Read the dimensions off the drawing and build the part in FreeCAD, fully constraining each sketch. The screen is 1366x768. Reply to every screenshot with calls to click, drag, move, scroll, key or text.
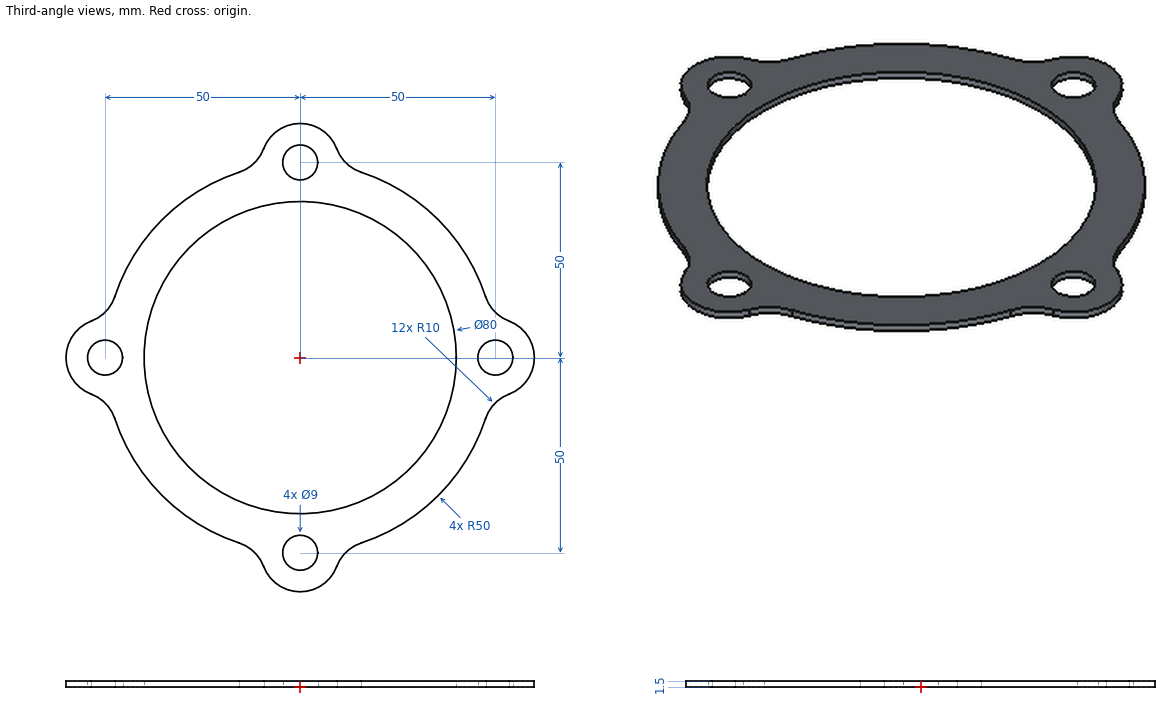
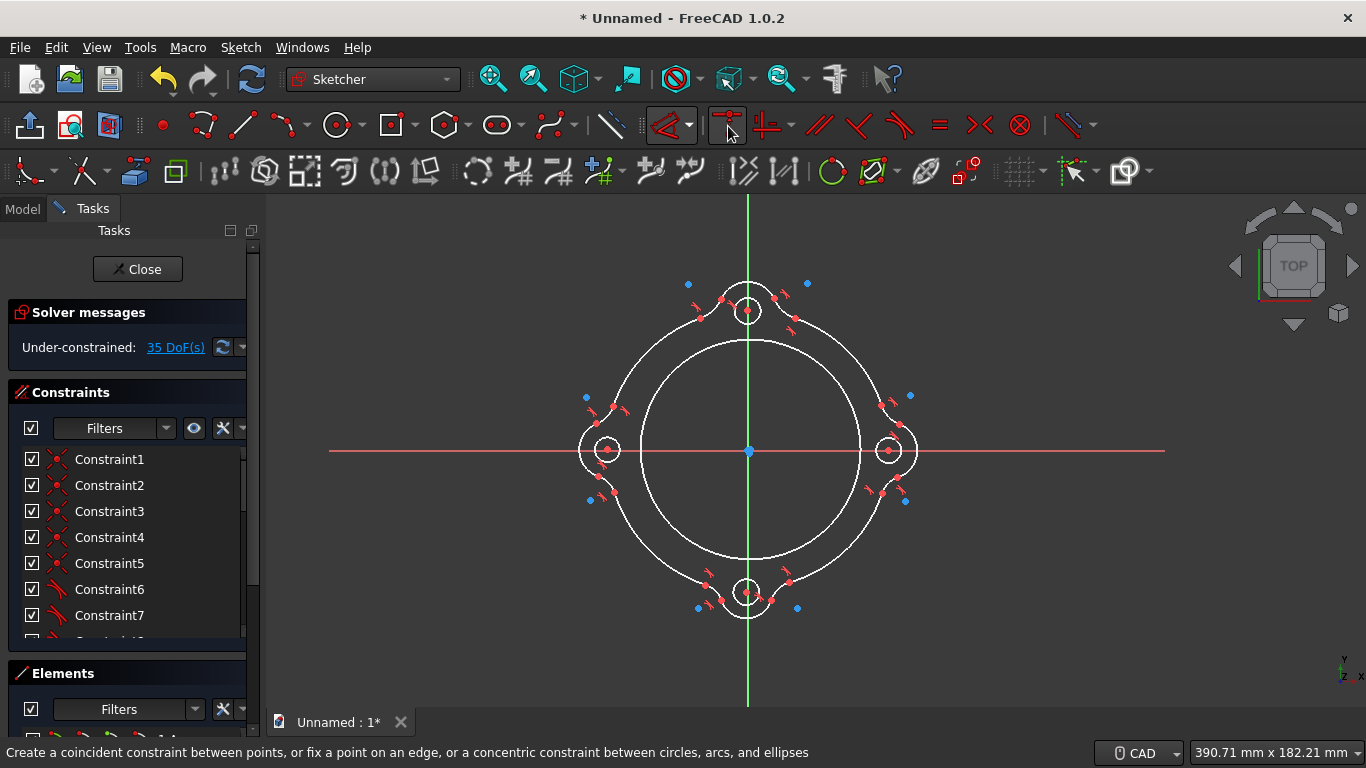
click(828, 371)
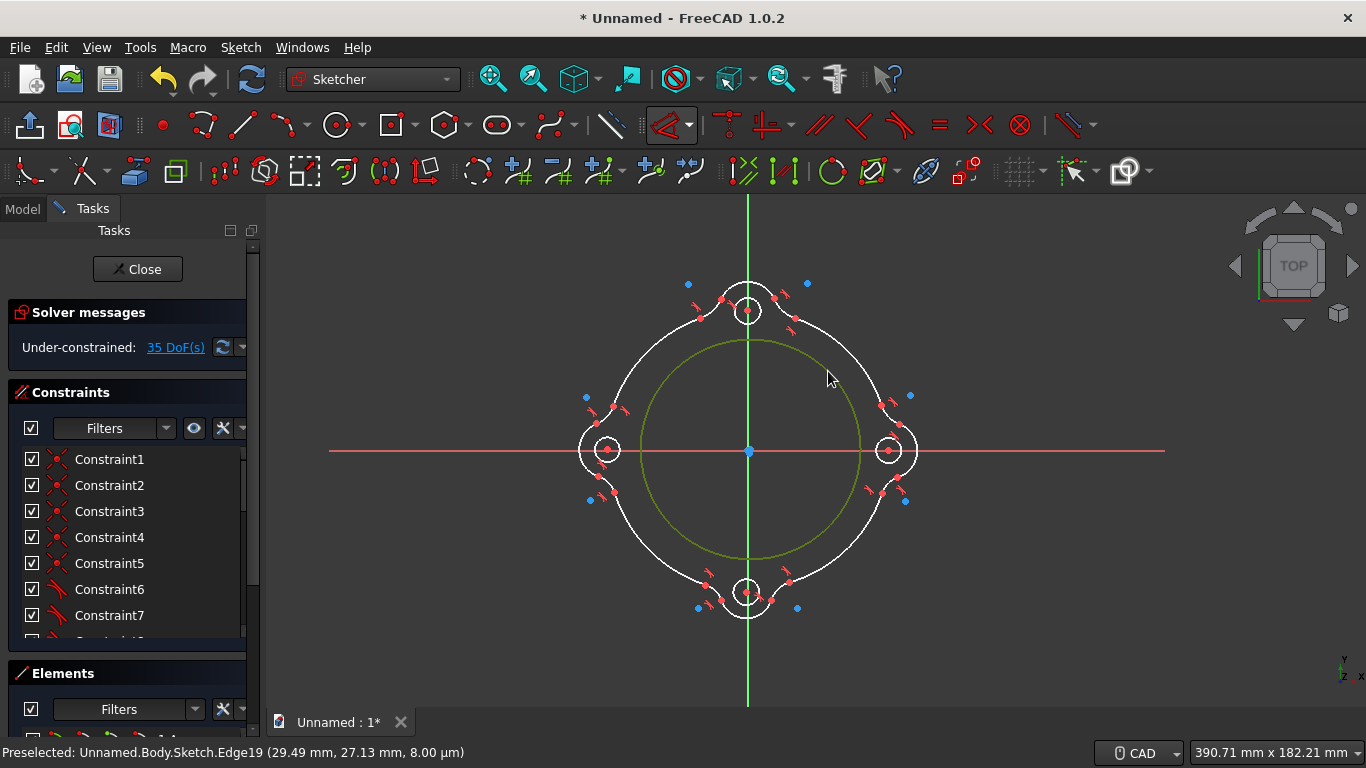
click(865, 371)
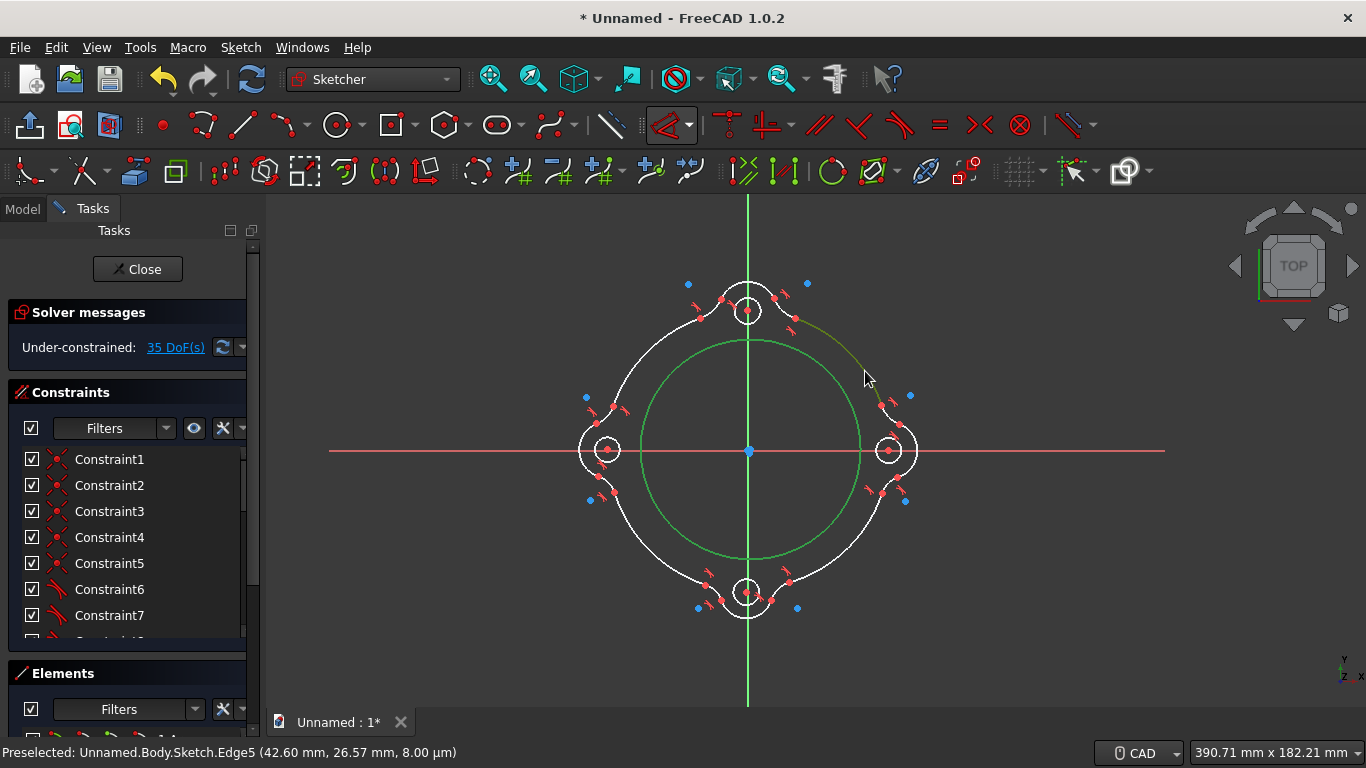
click(728, 126)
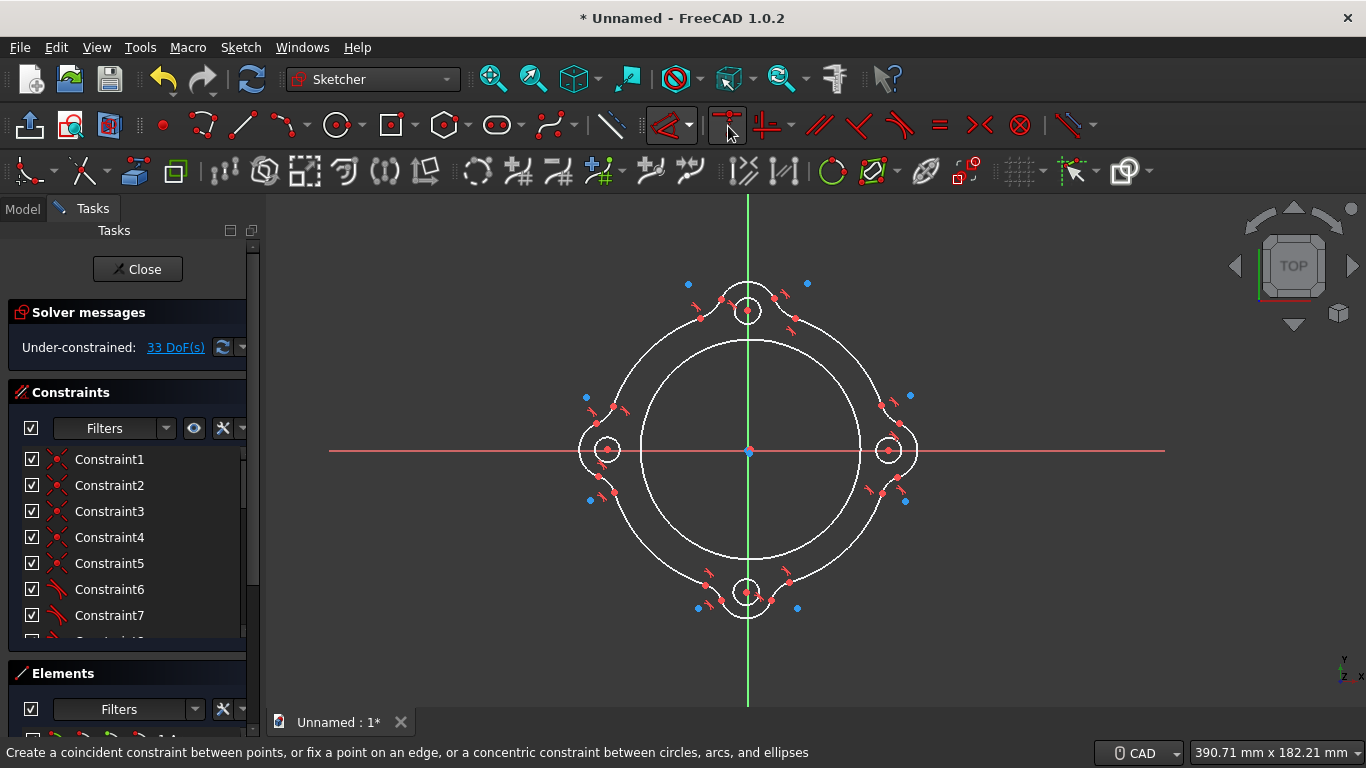
click(828, 371)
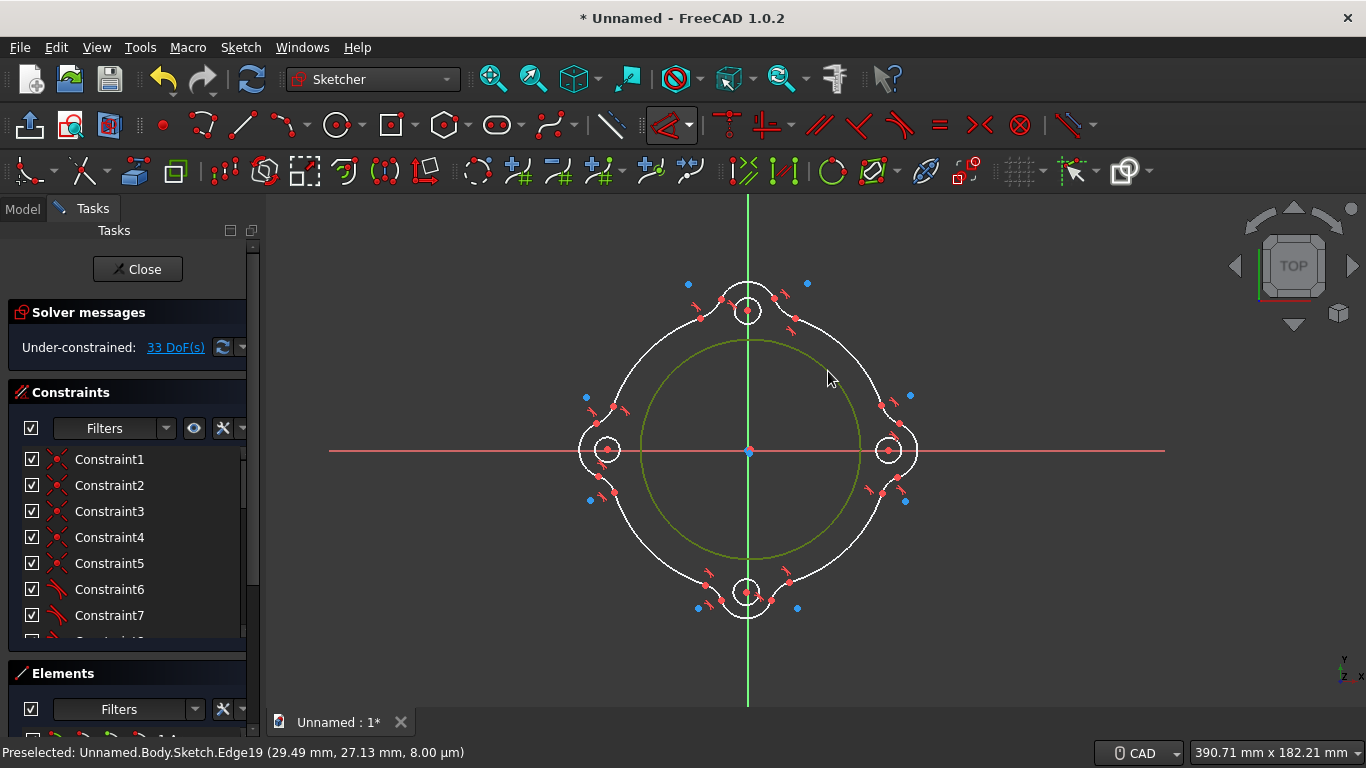
click(666, 336)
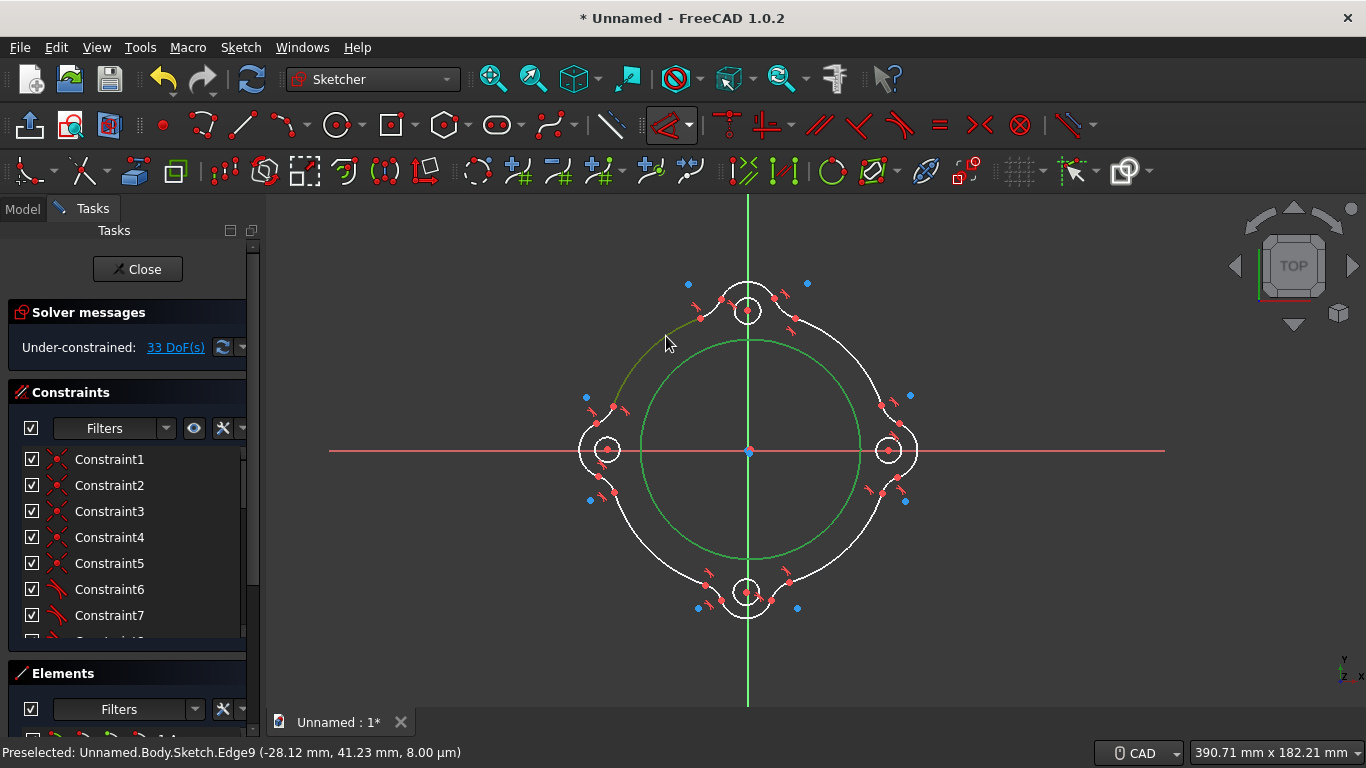
click(728, 126)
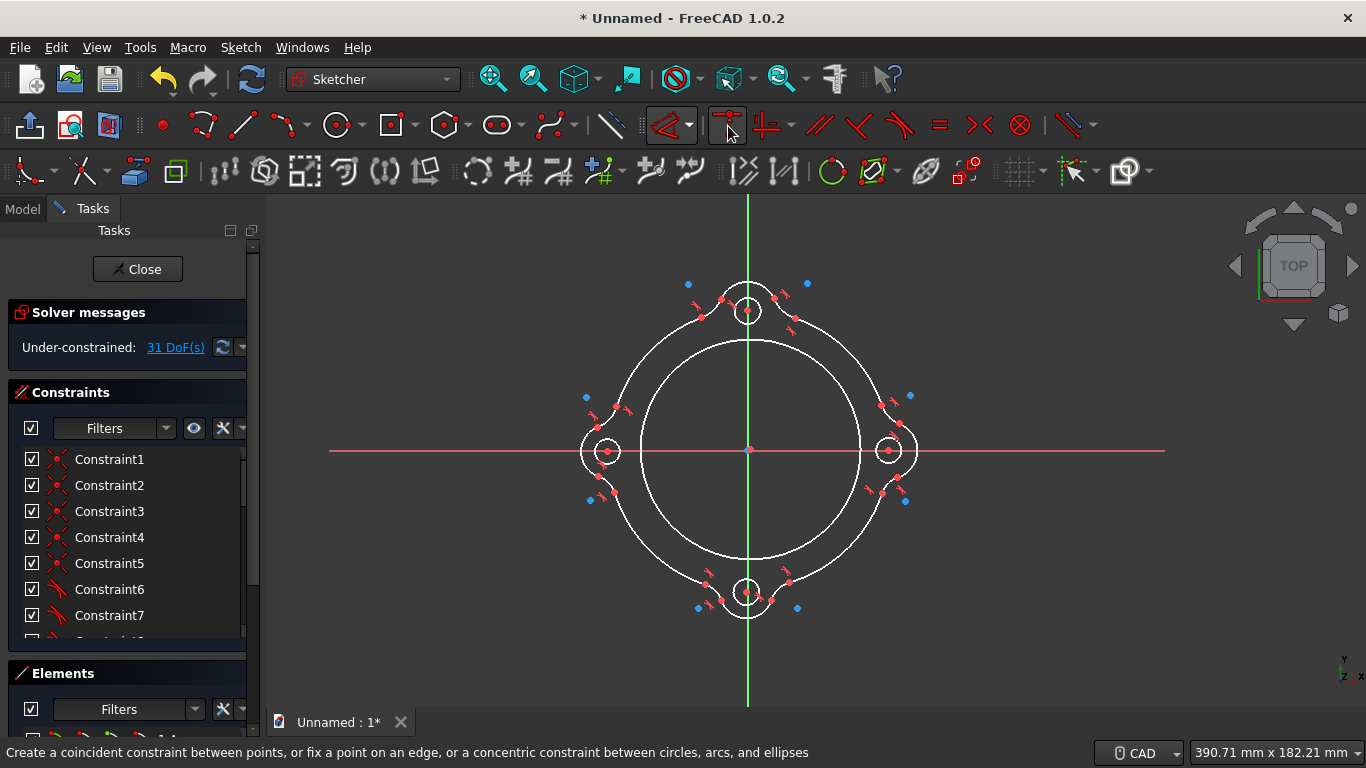
scroll(749, 450, up, 6)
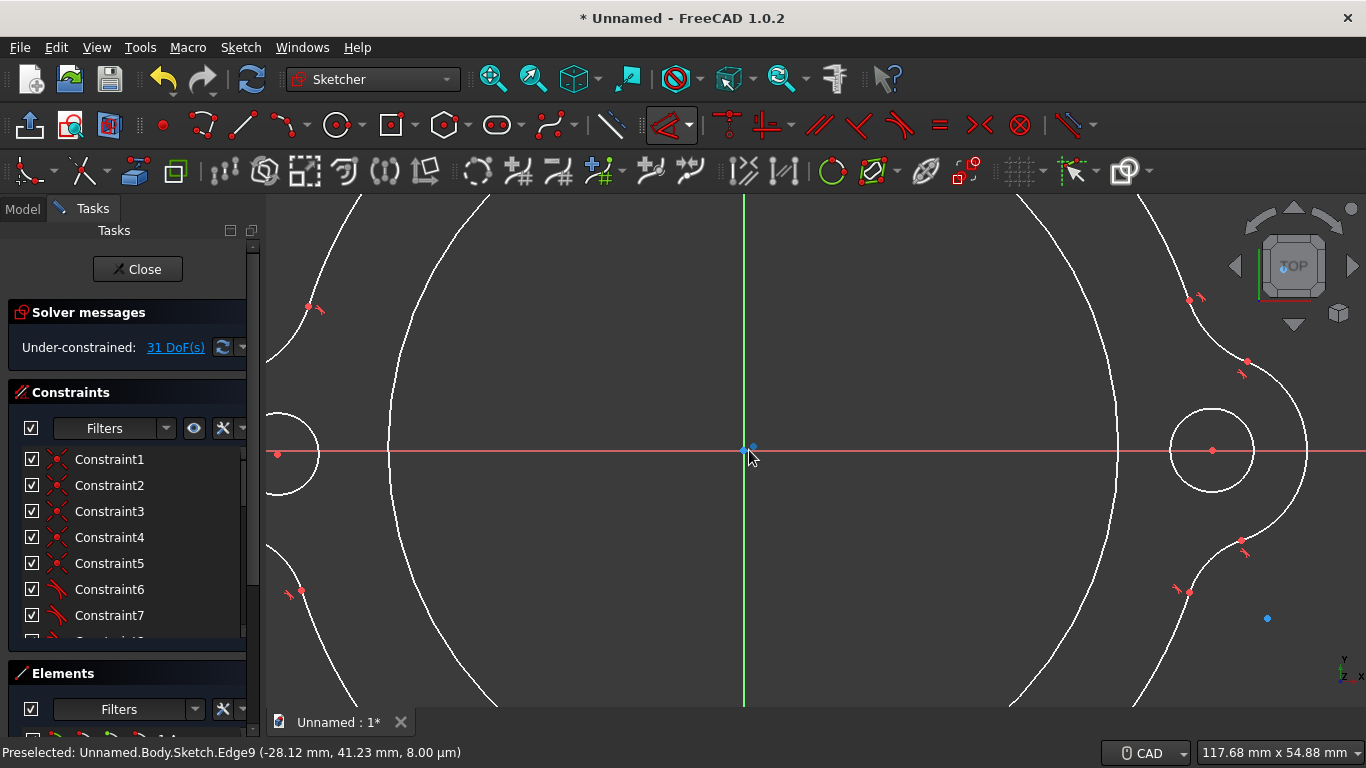
drag(734, 437, 763, 461)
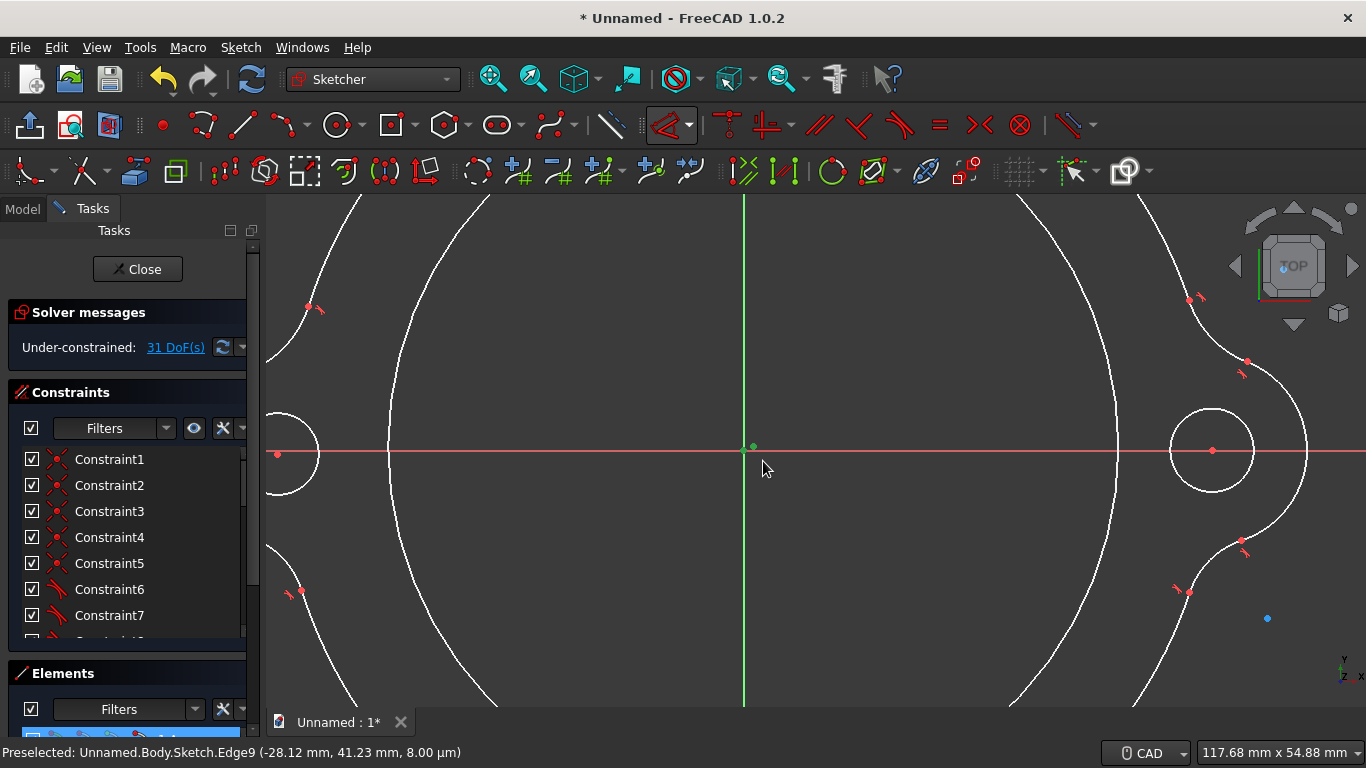
click(728, 126)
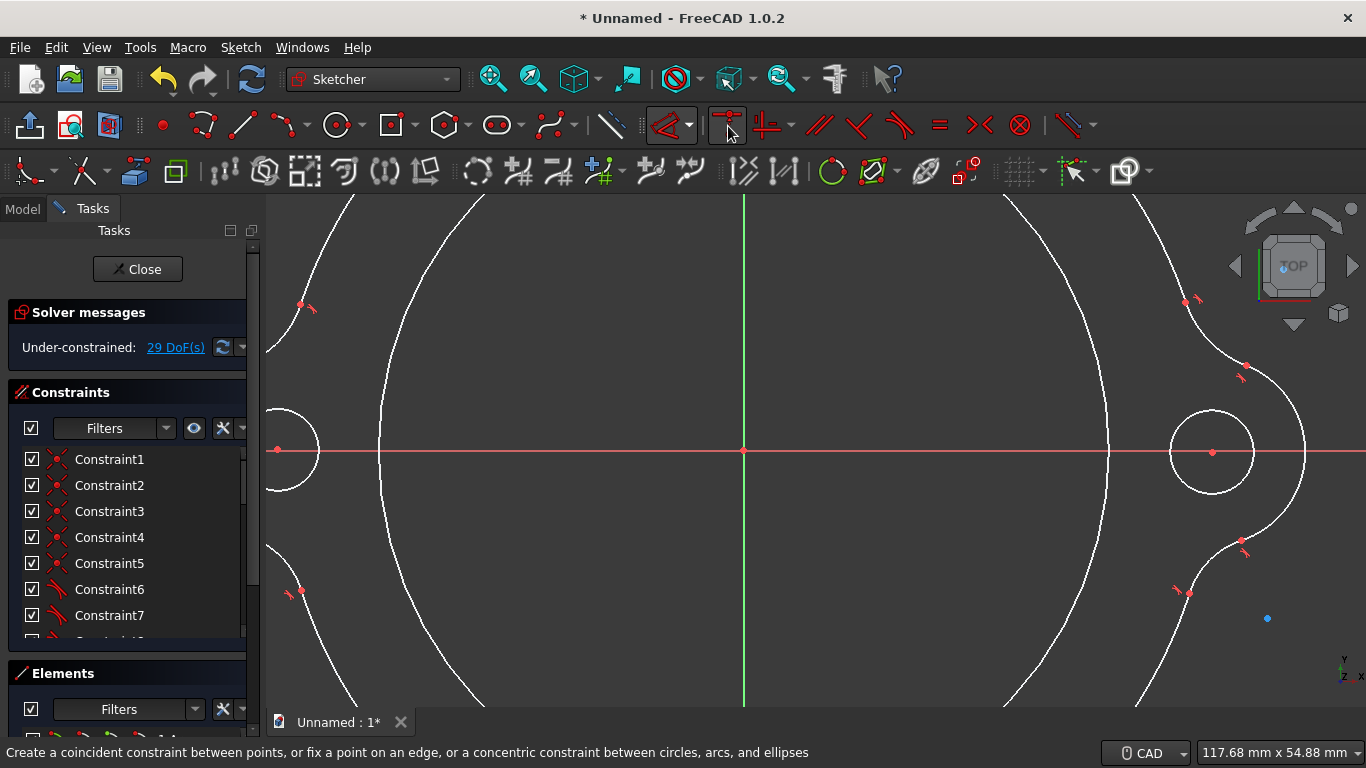
click(1200, 572)